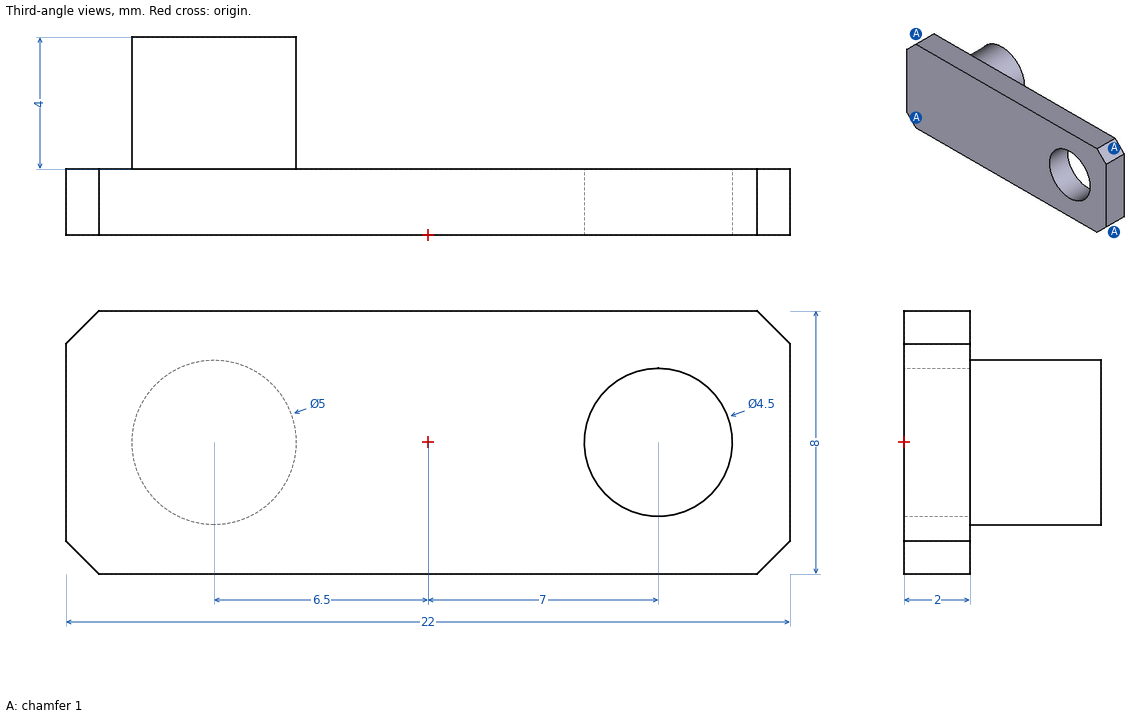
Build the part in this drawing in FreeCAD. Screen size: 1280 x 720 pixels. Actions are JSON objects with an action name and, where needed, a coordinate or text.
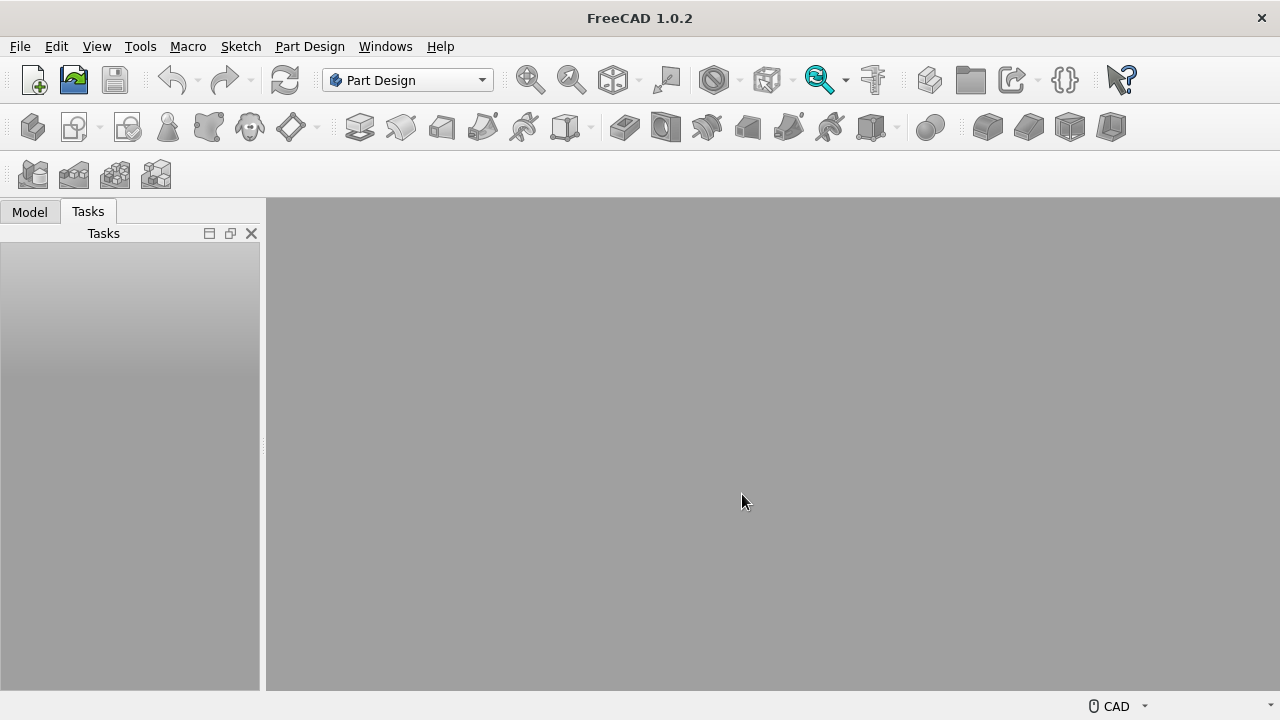
{"action": "left_click", "coordinate": [33, 80]}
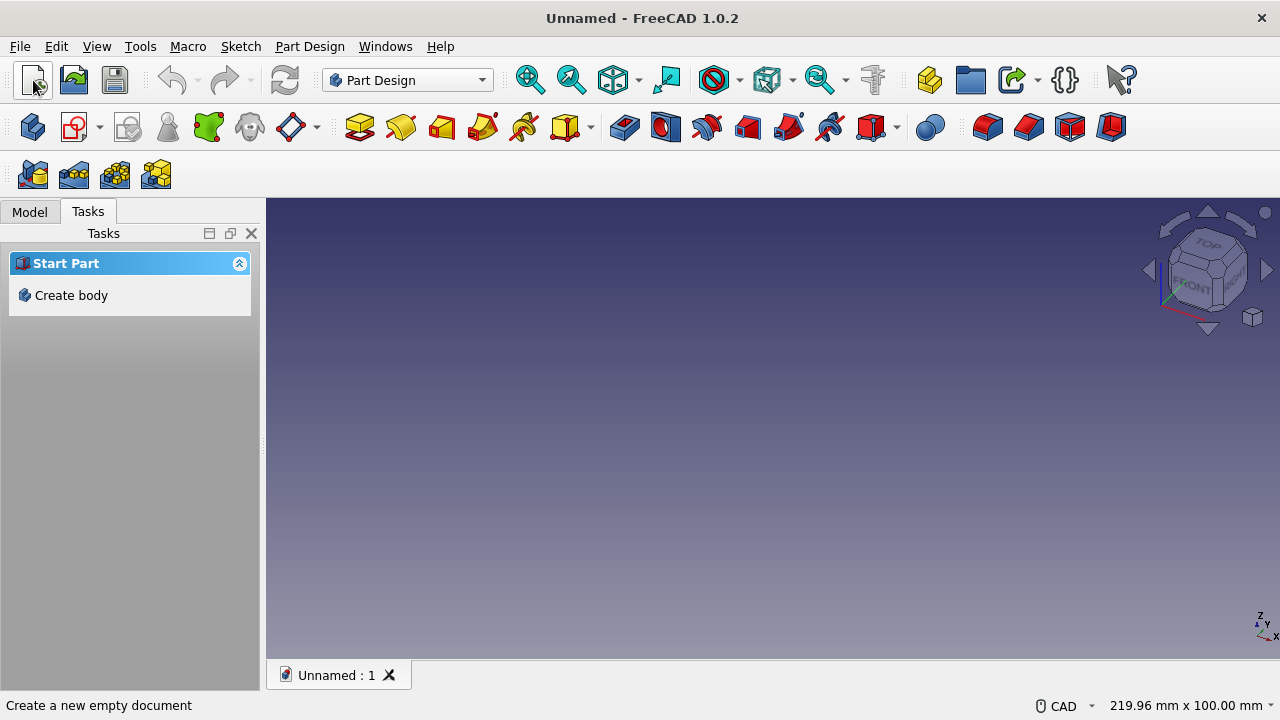
{"action": "left_click", "coordinate": [74, 128]}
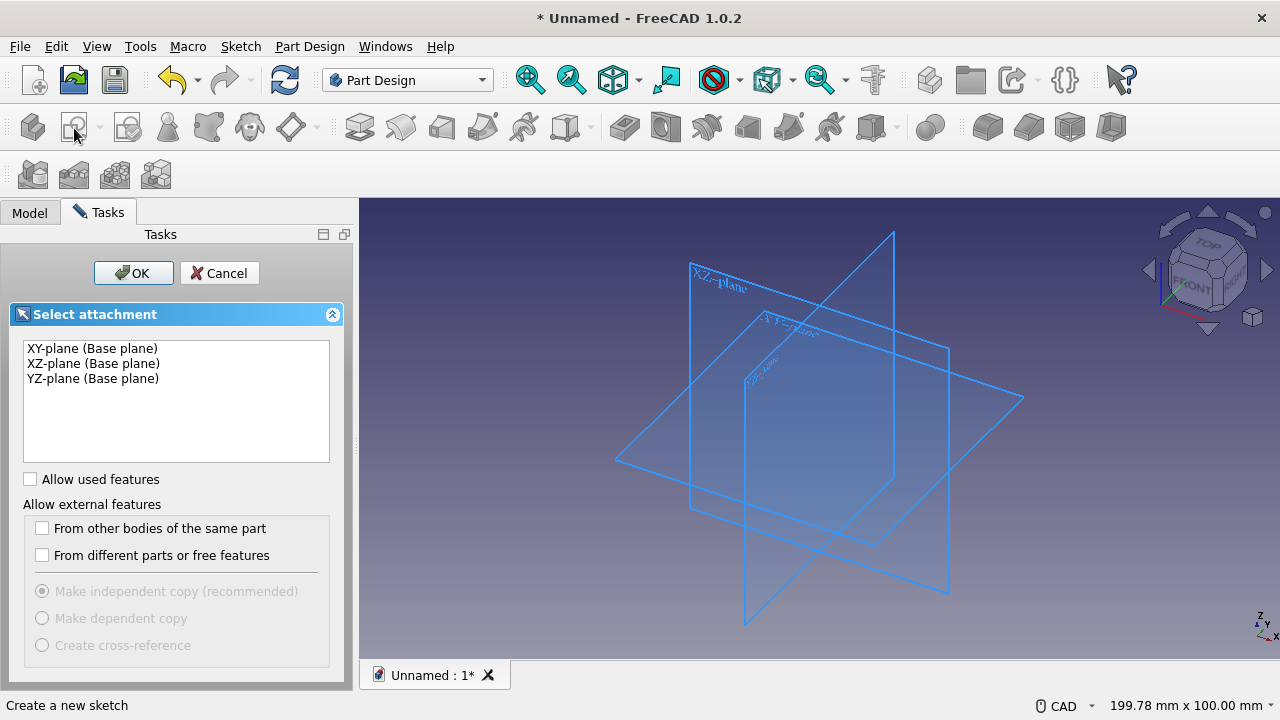
{"action": "left_click", "coordinate": [84, 364]}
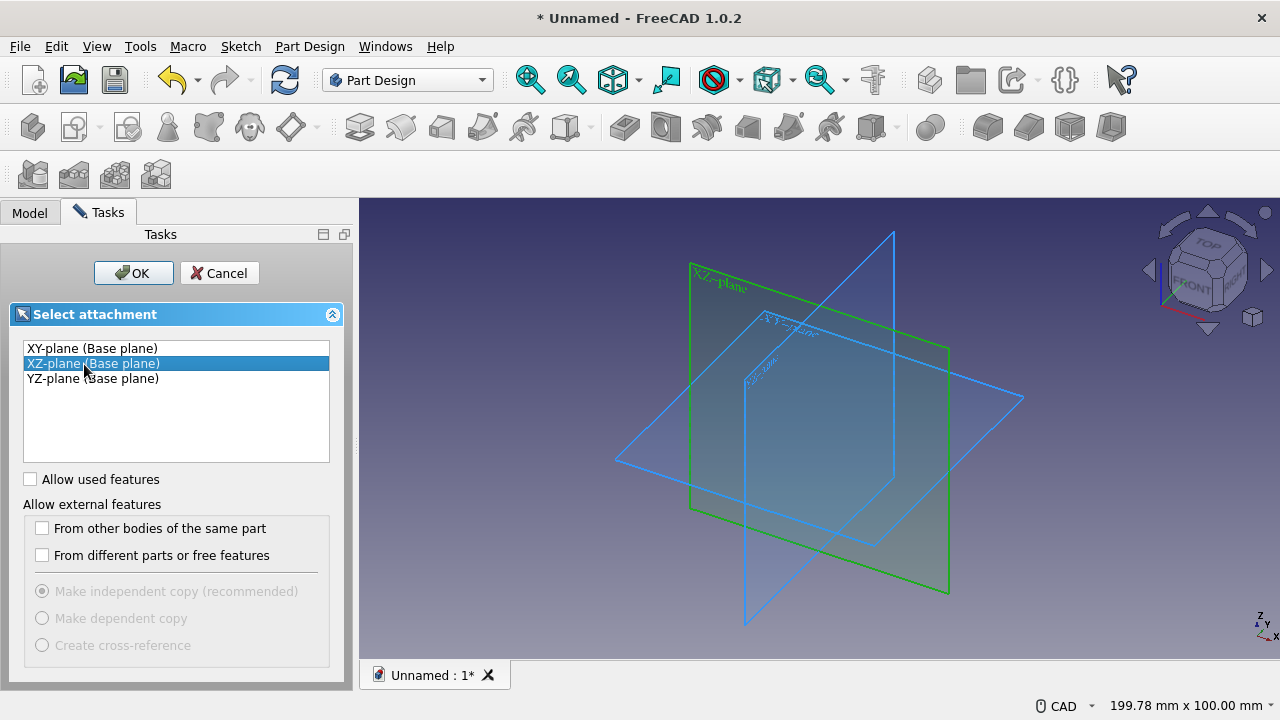
{"action": "left_click", "coordinate": [134, 273]}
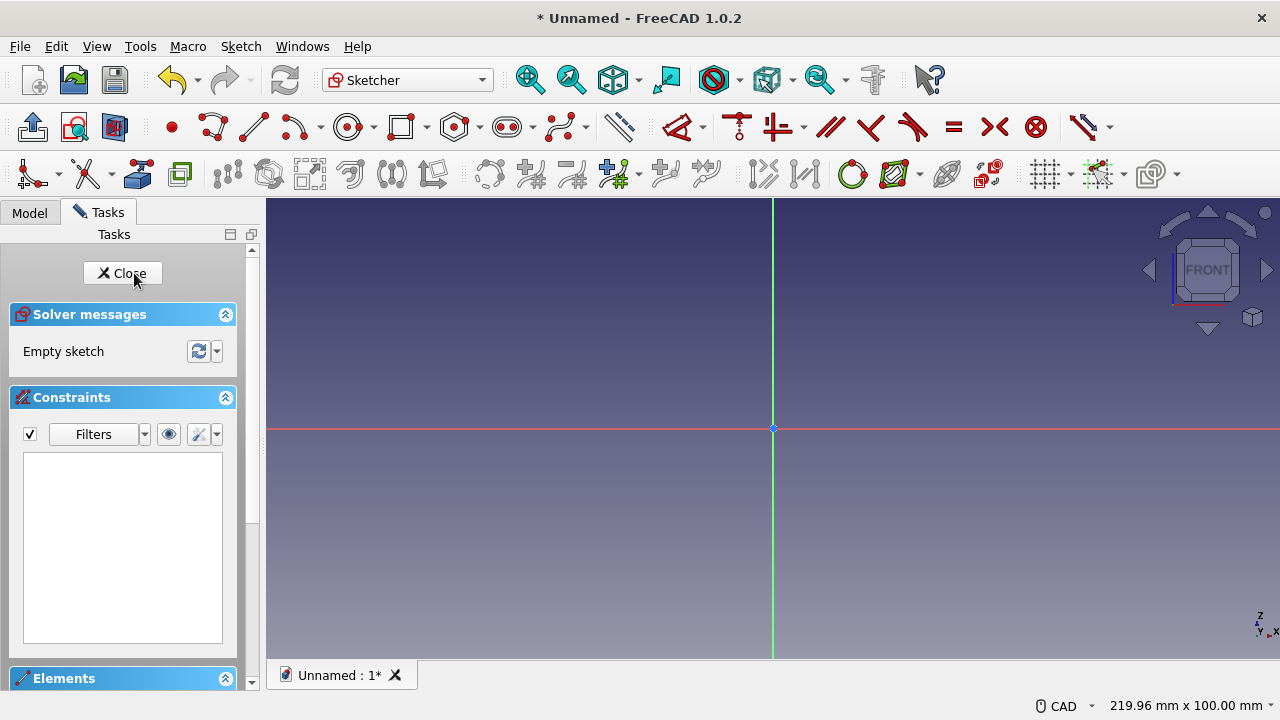
{"action": "scroll", "coordinate": [787, 428], "scroll_direction": "up", "scroll_amount": 9}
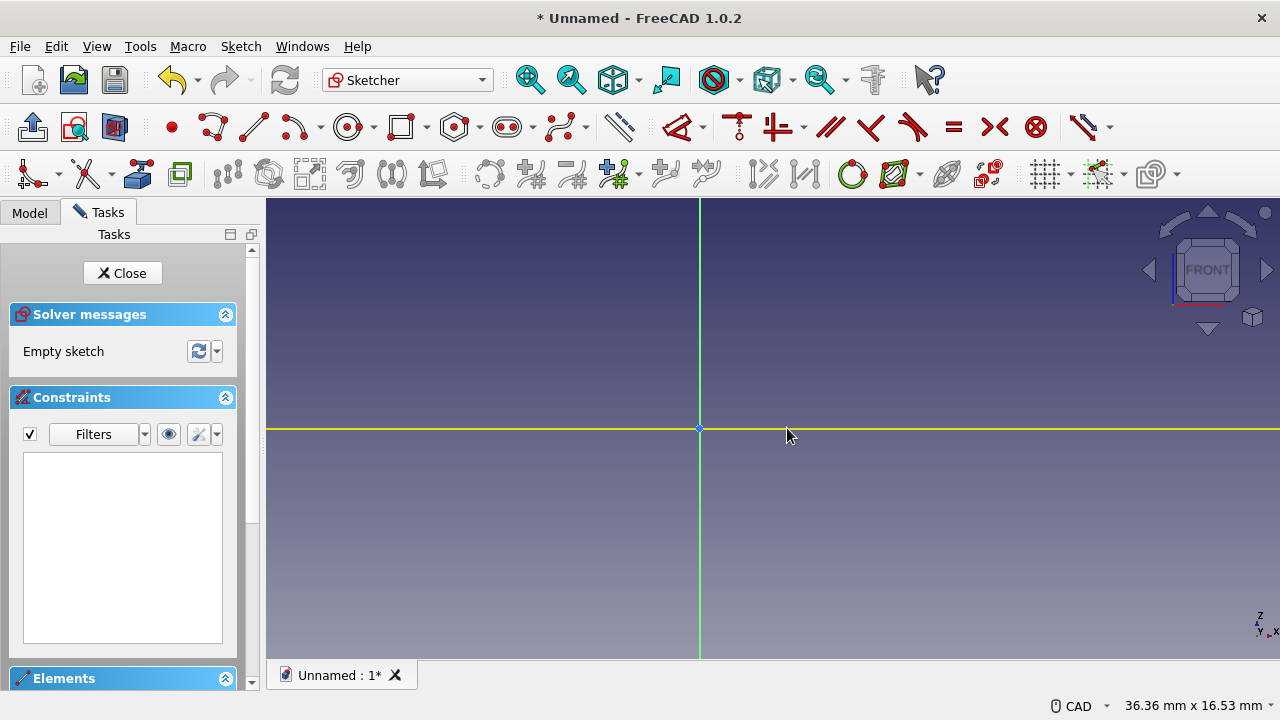
{"action": "left_click", "coordinate": [426, 128]}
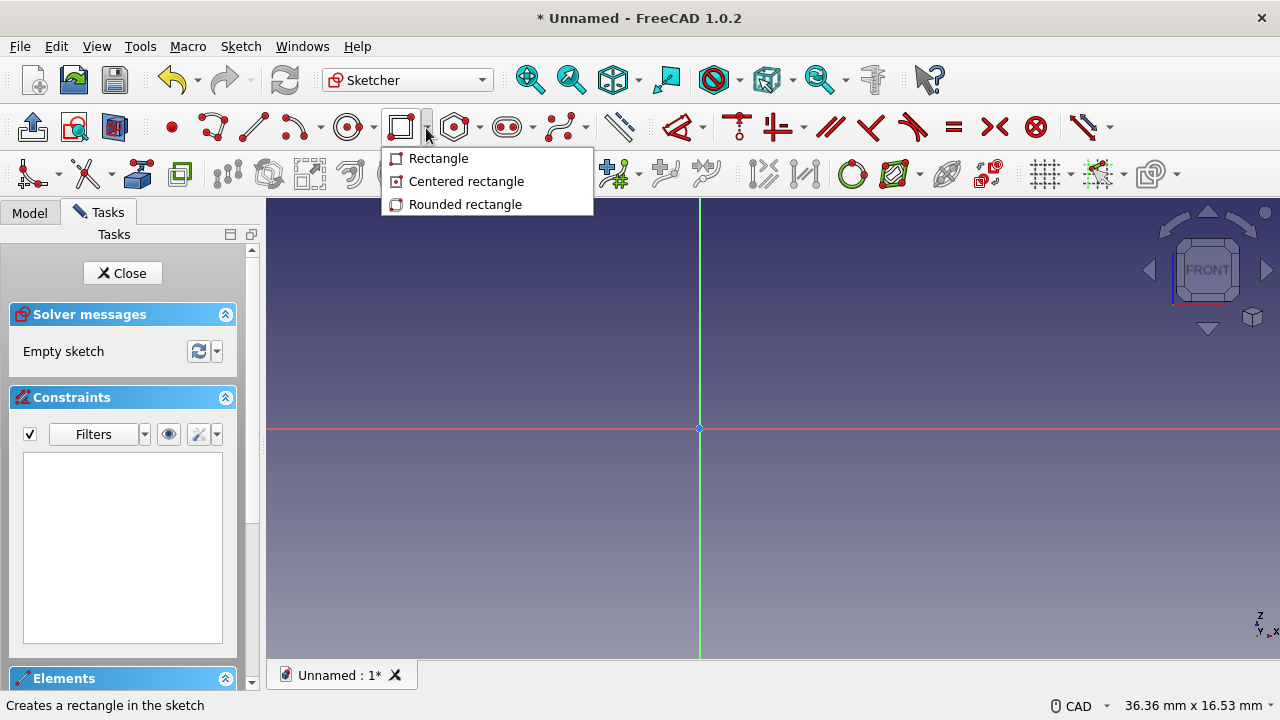
{"action": "left_click", "coordinate": [488, 182]}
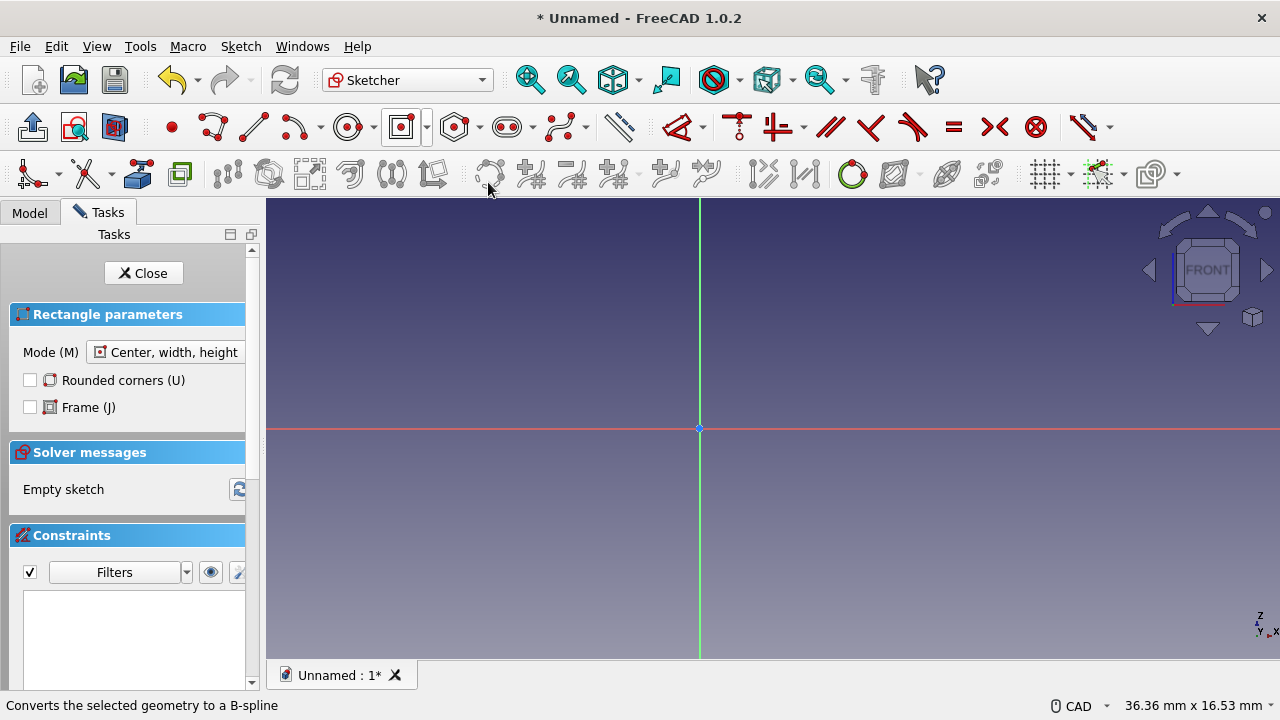
{"action": "left_click", "coordinate": [700, 428]}
{"action": "left_click", "coordinate": [1006, 317]}
{"action": "key", "text": "Escape"}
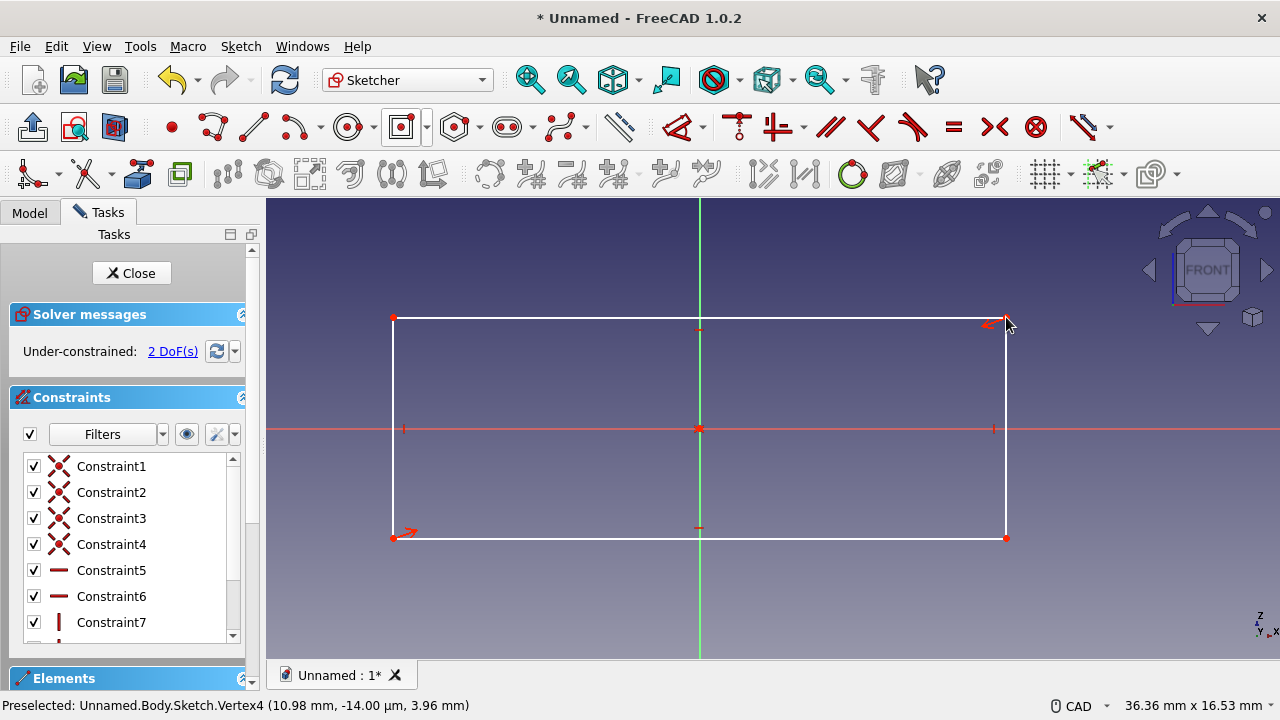
{"action": "left_click", "coordinate": [676, 128]}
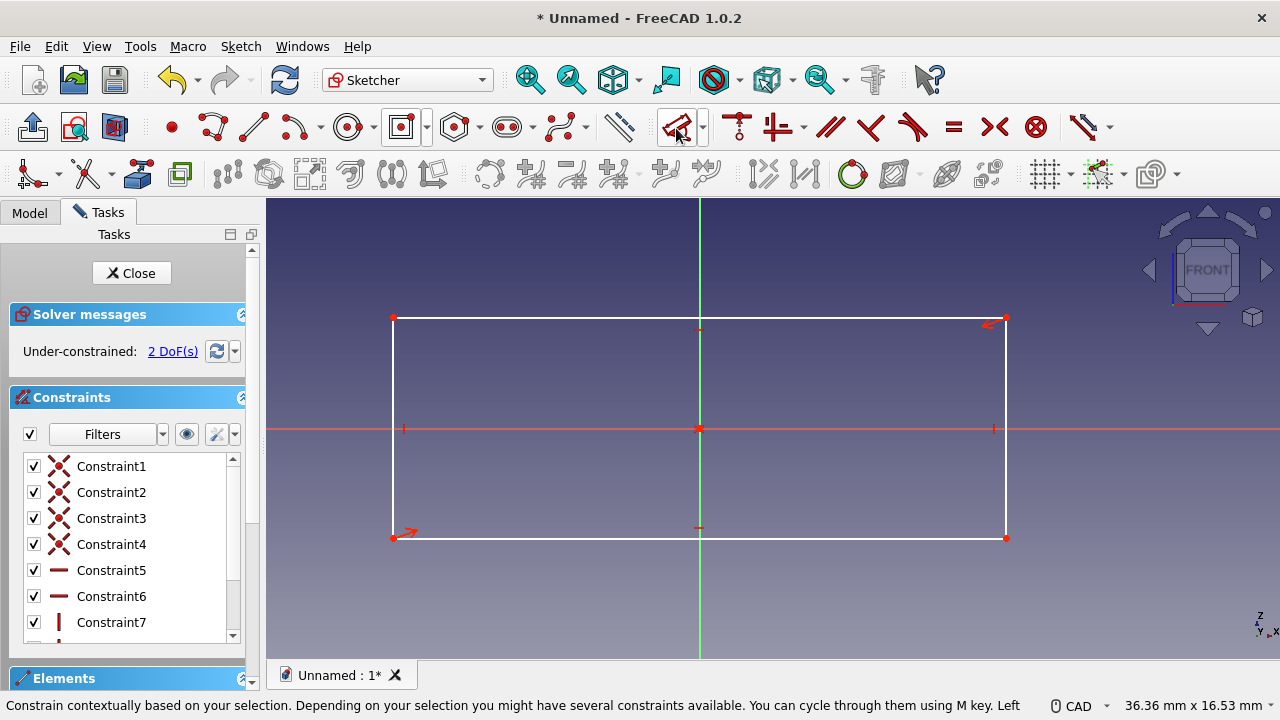
{"action": "left_click", "coordinate": [1006, 473]}
{"action": "left_click", "coordinate": [1040, 378]}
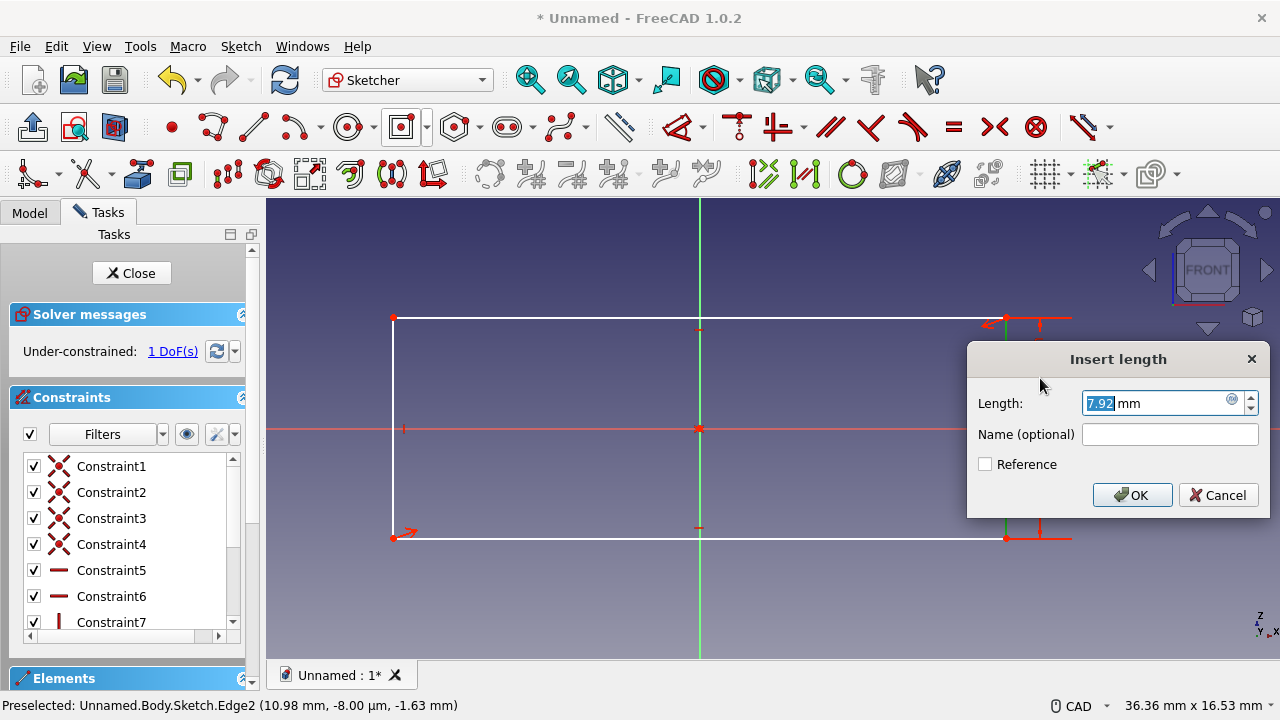
{"action": "type", "text": "8"}
{"action": "key", "text": "Return"}